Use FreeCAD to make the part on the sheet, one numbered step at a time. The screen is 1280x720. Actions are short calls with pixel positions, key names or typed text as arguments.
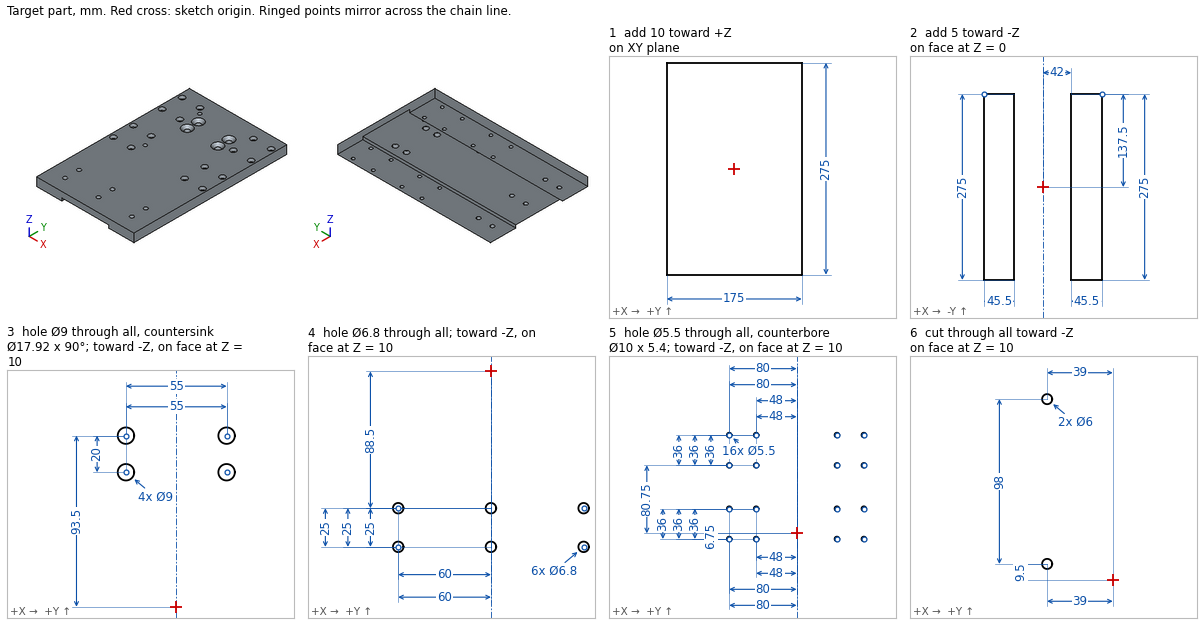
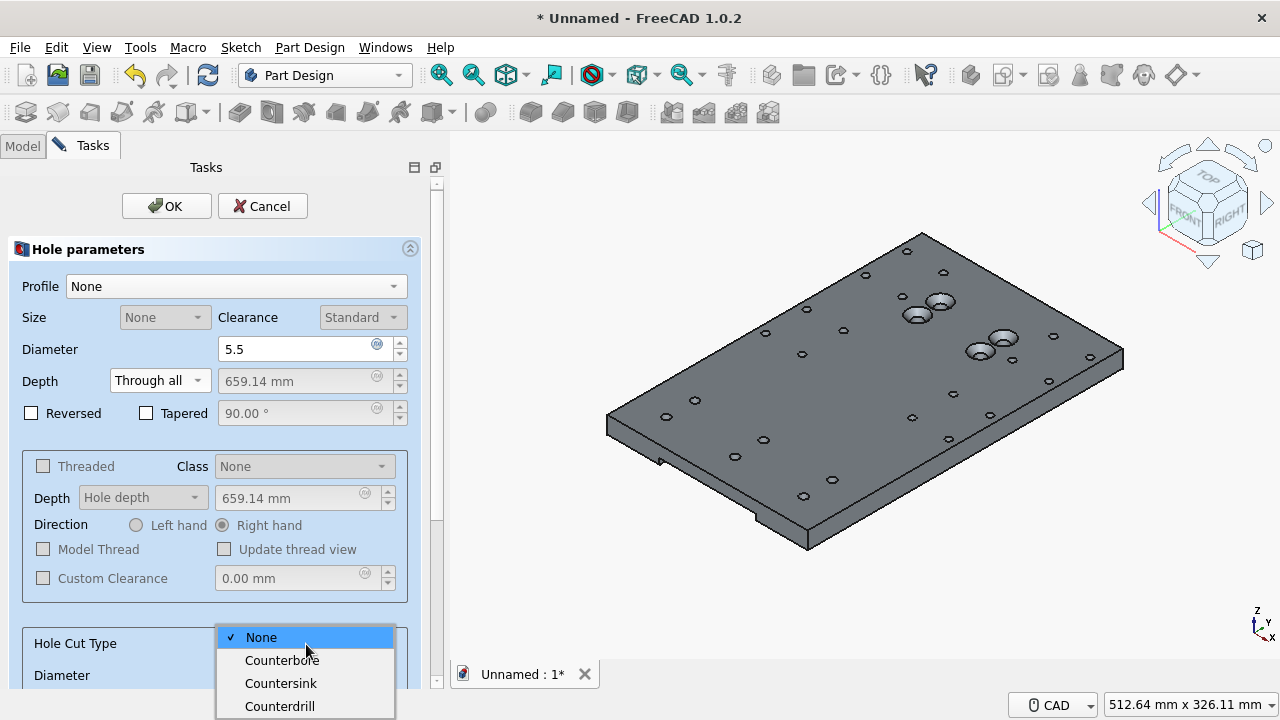
click(304, 660)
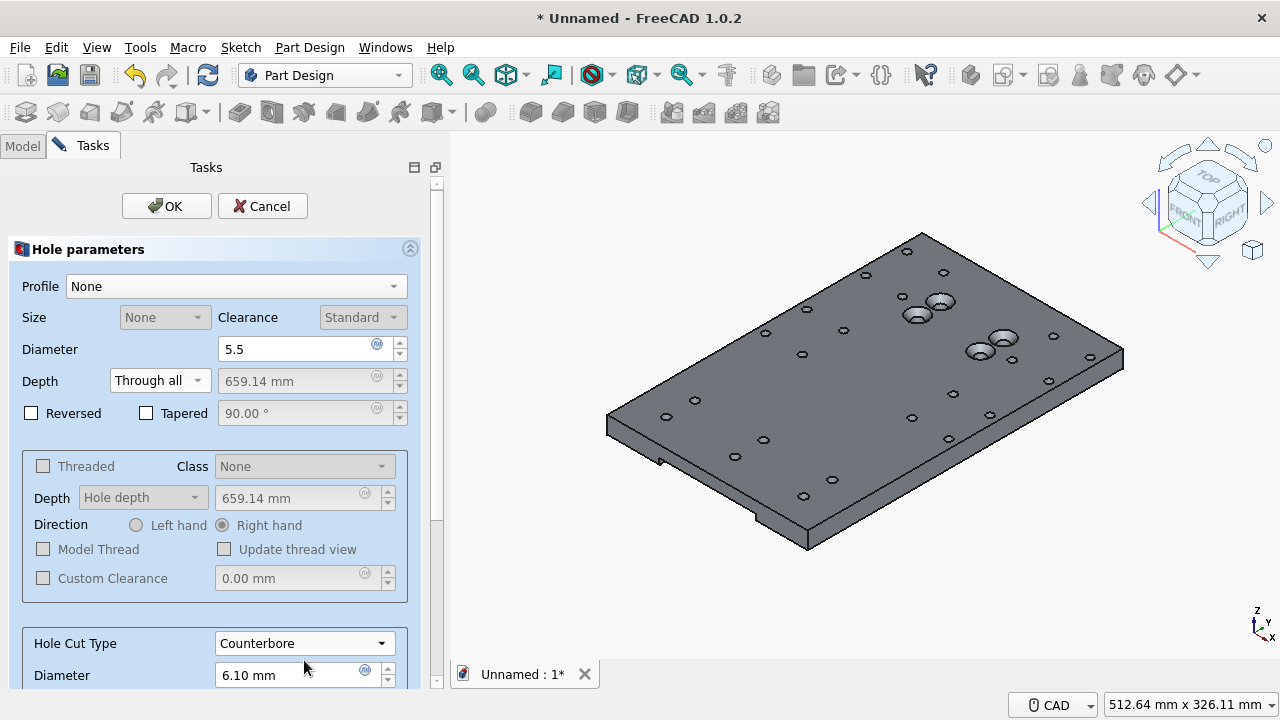
triple_click(298, 675)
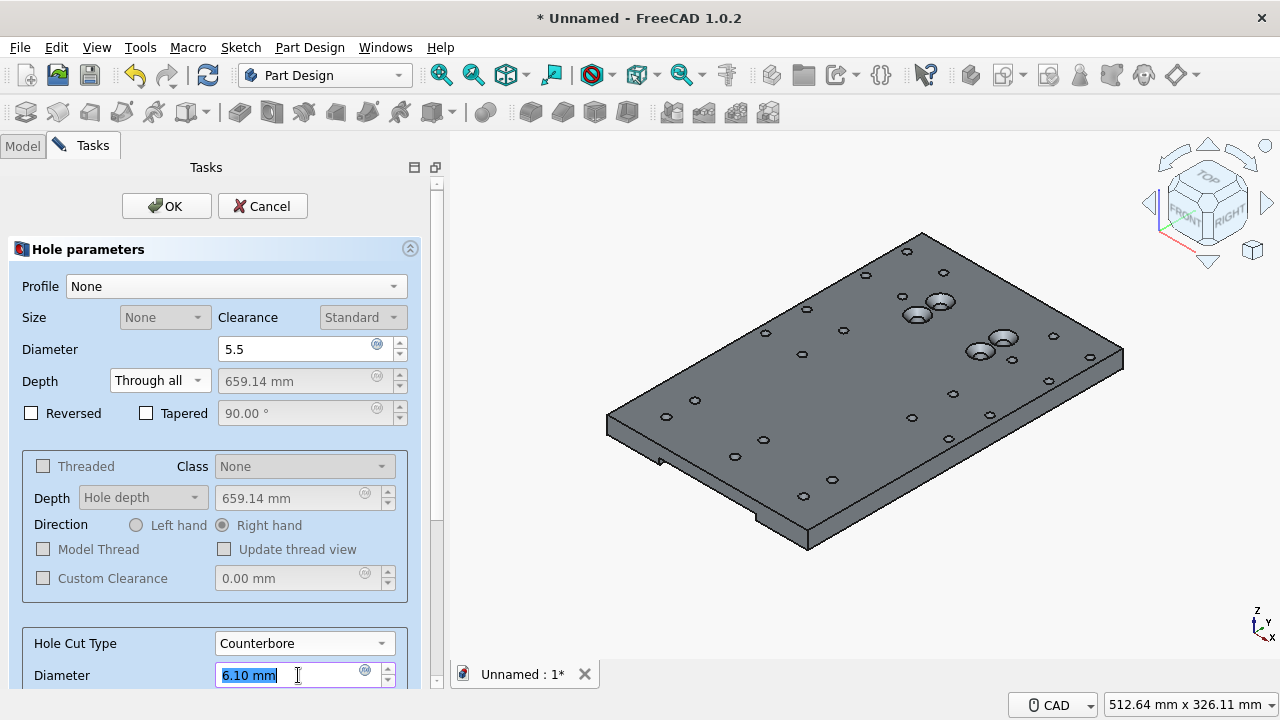
text(10)
key(Tab)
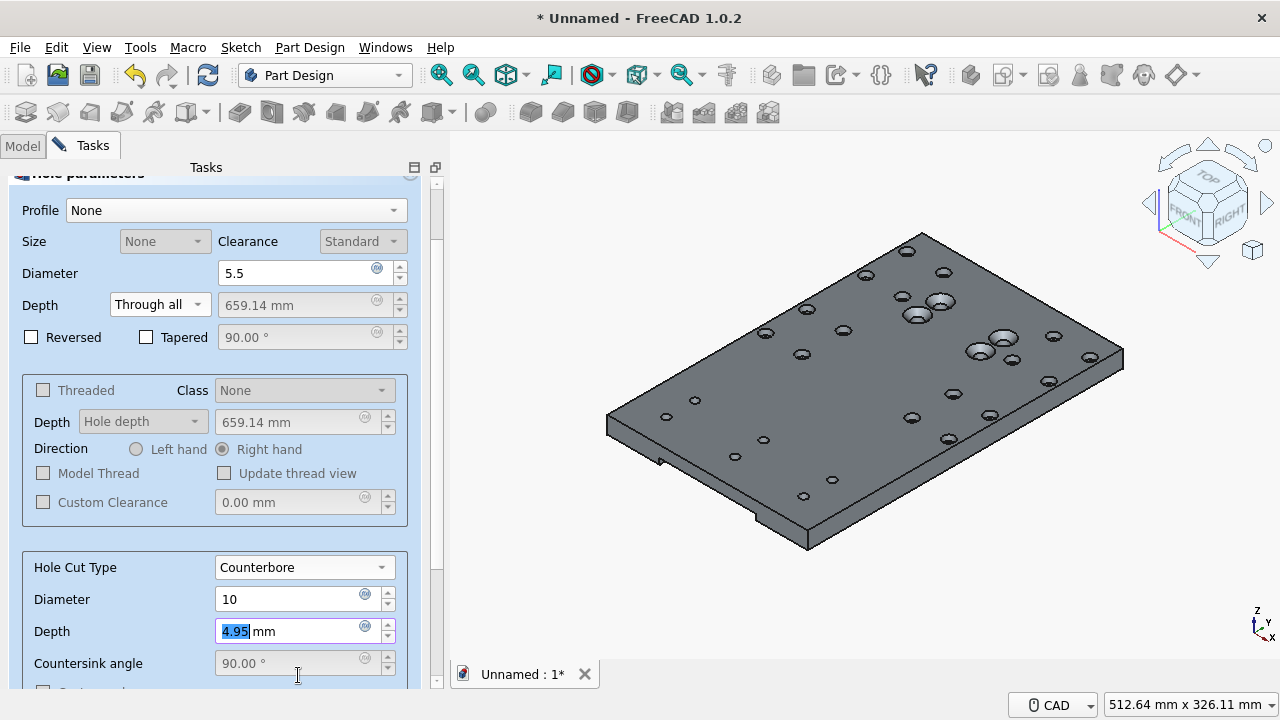
text(5.4)
key(Tab)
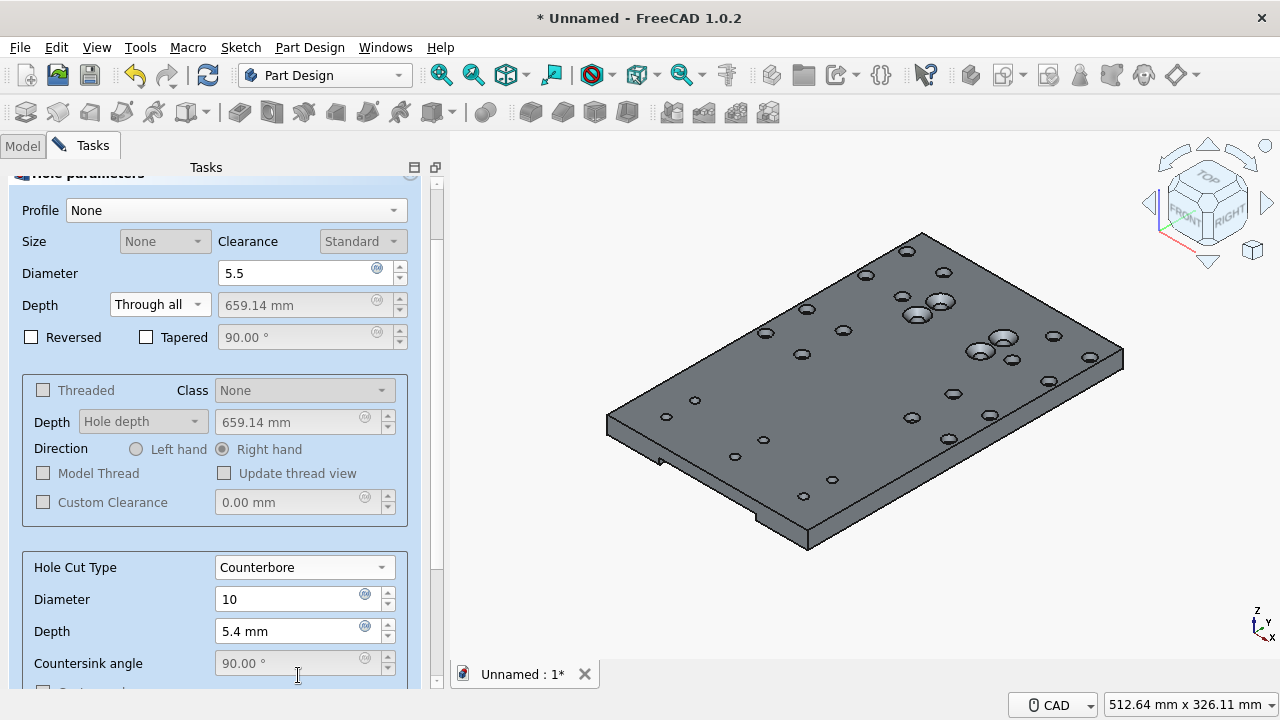
scroll(437, 432, up, 3)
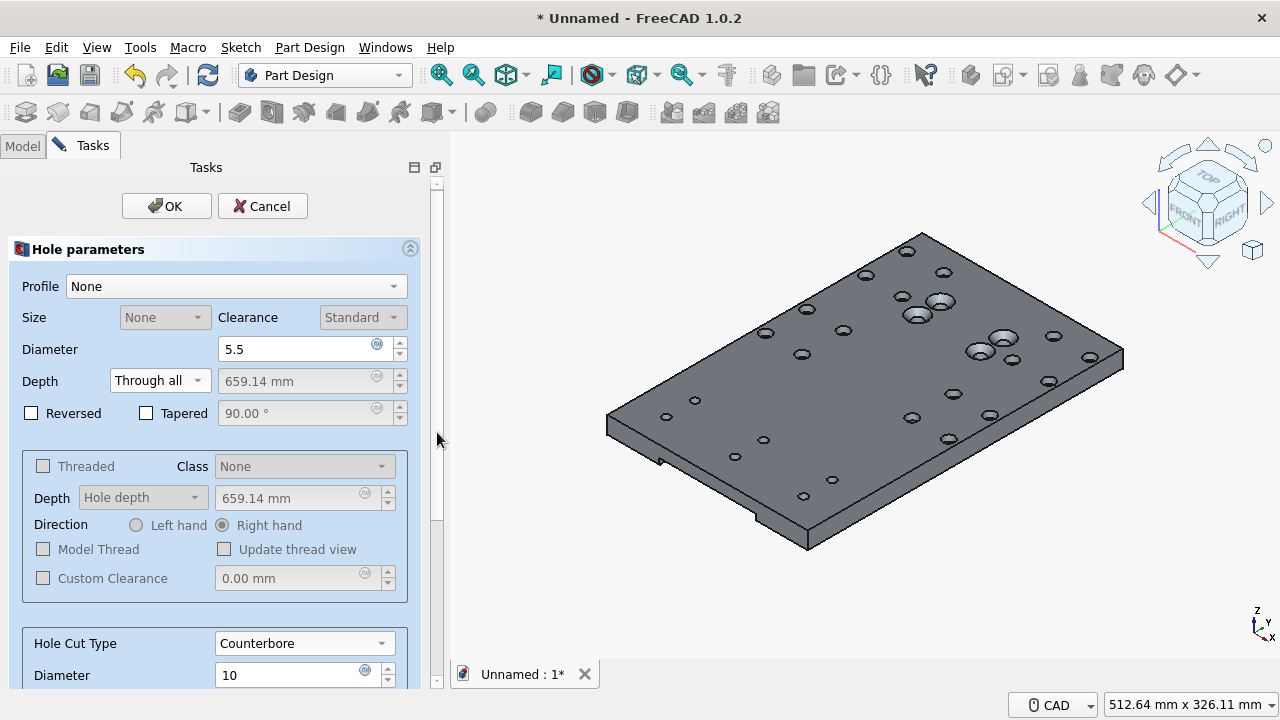
click(167, 206)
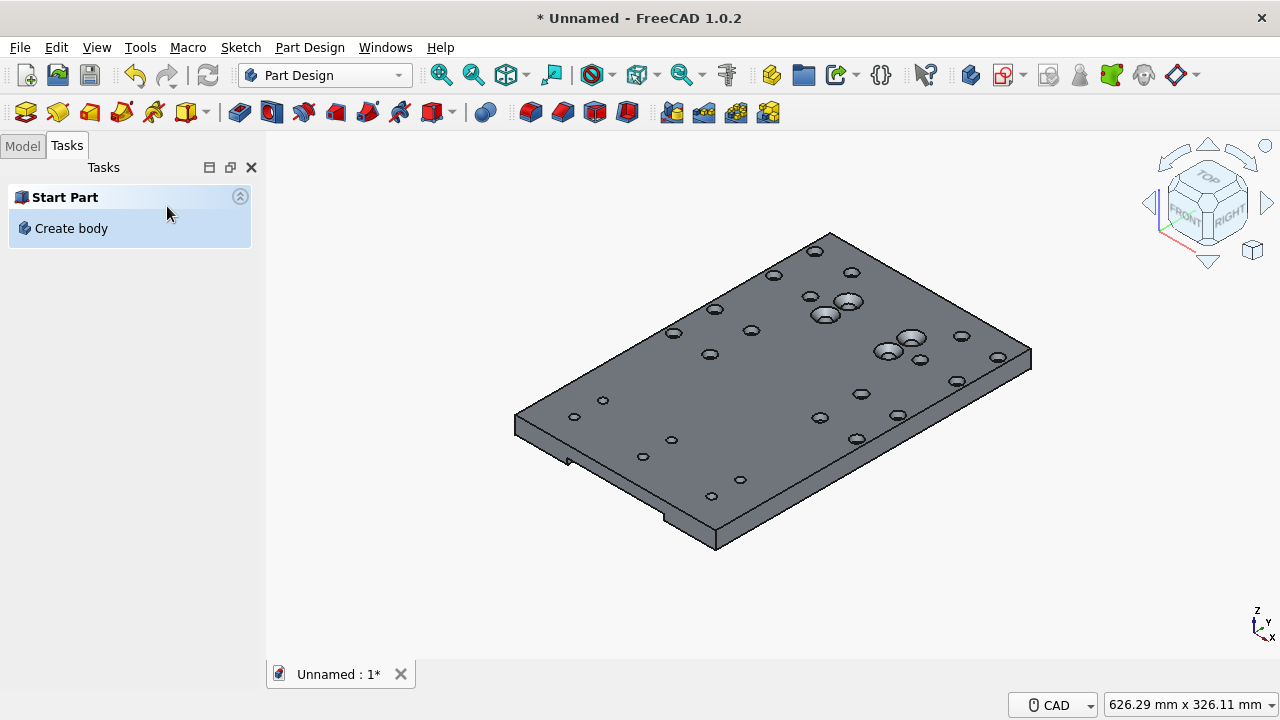
click(728, 407)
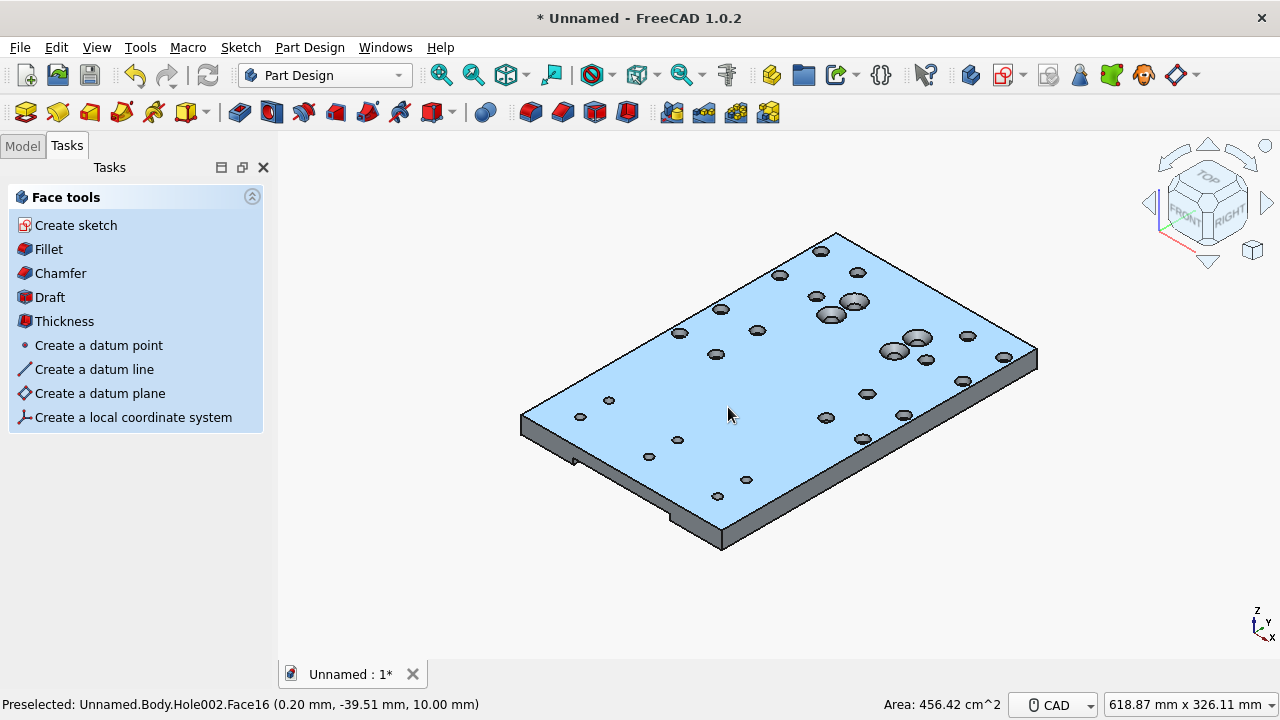
click(1004, 76)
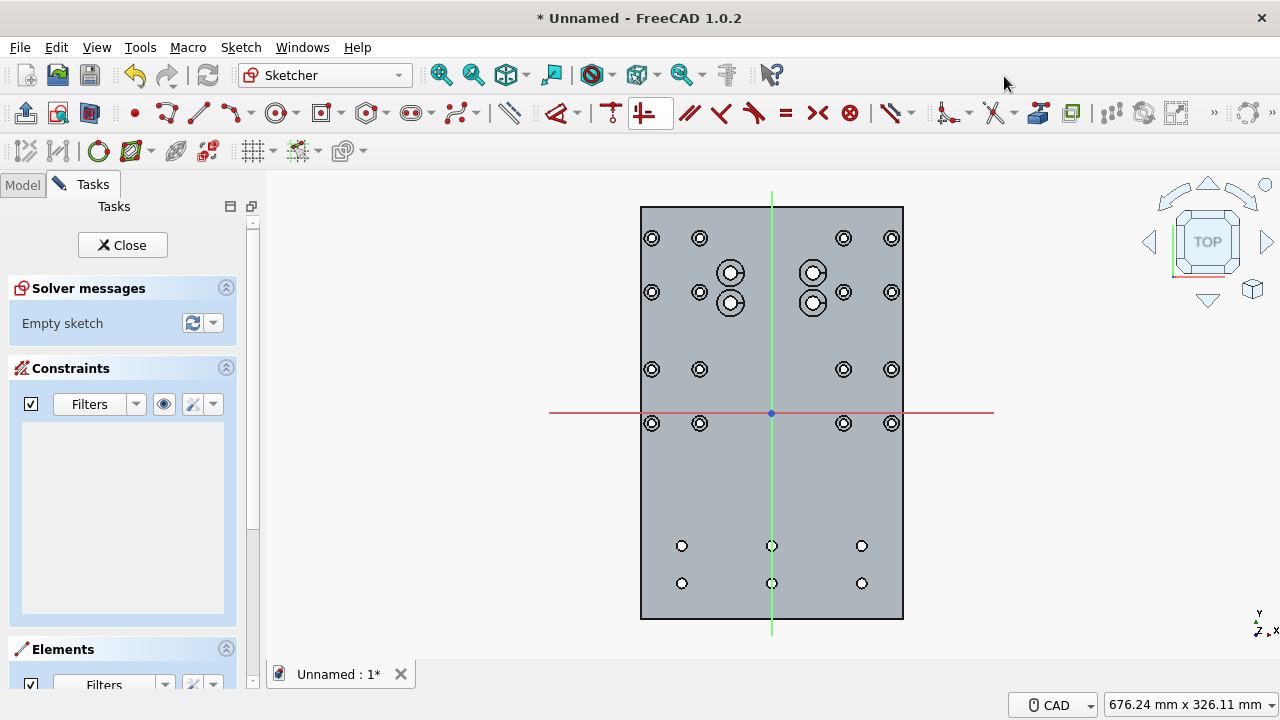
scroll(784, 228, up, 3)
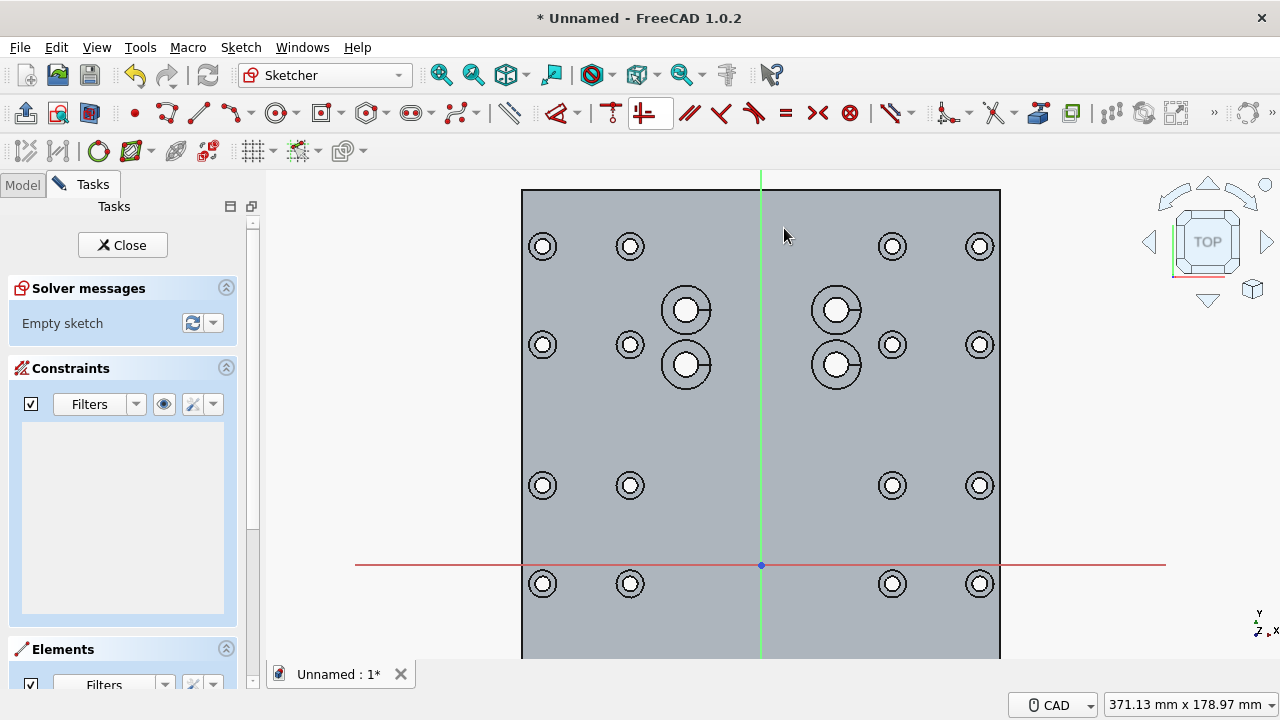
click(276, 114)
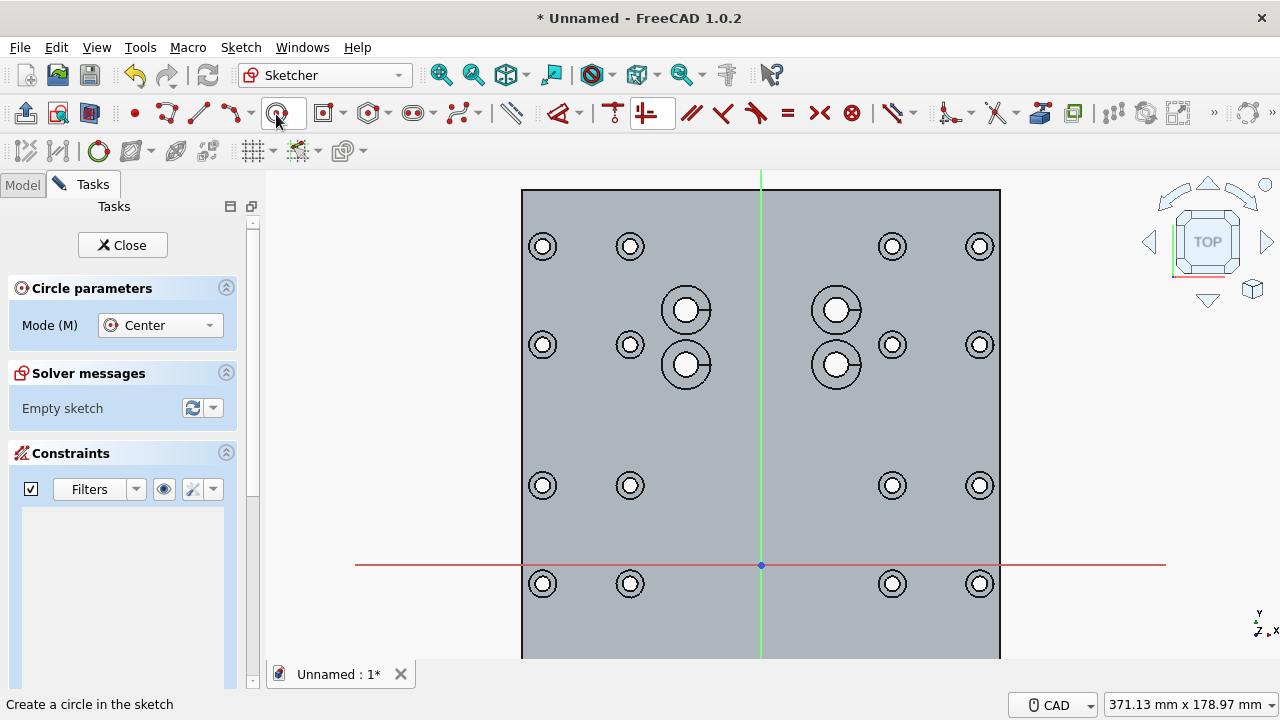
scroll(655, 272, up, 6)